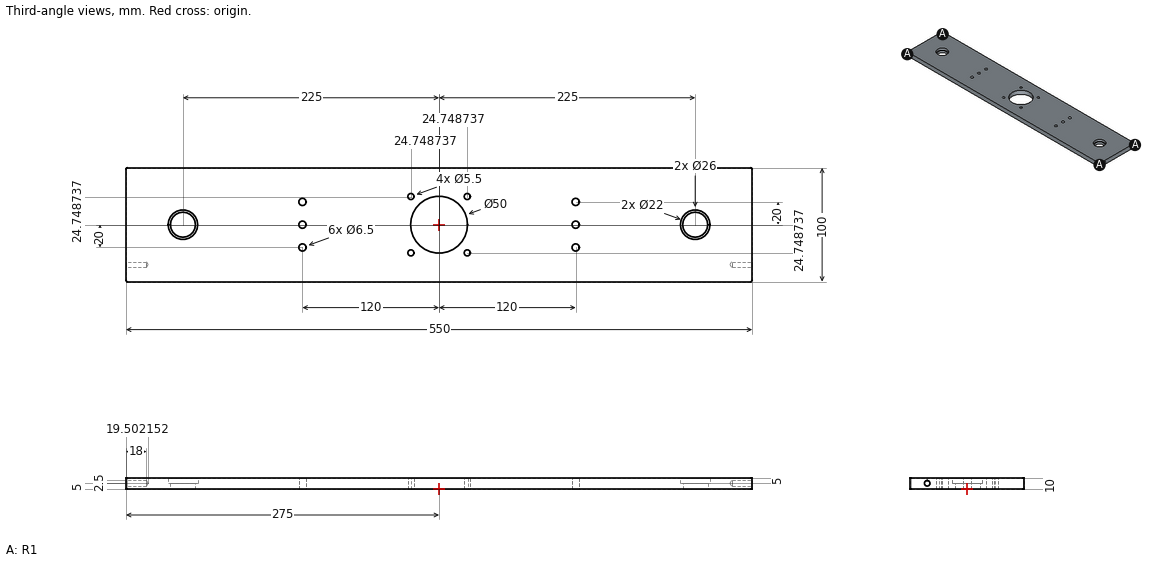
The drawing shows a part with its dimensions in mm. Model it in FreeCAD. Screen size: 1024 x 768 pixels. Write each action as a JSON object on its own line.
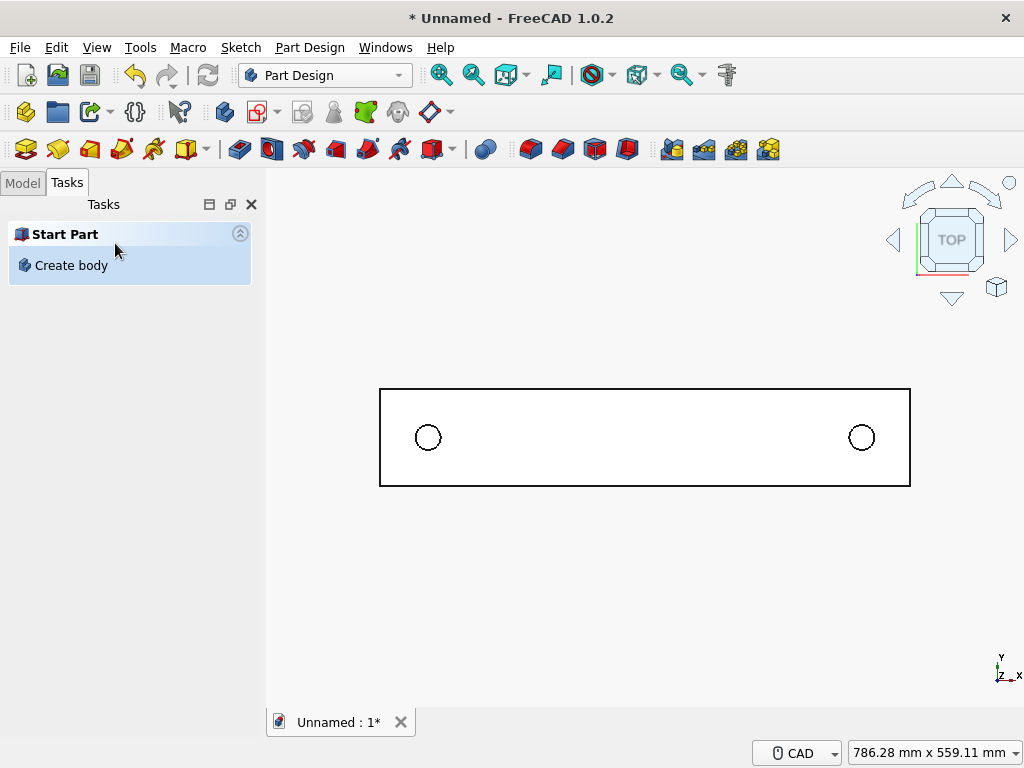
{"action": "left_click", "coordinate": [428, 437]}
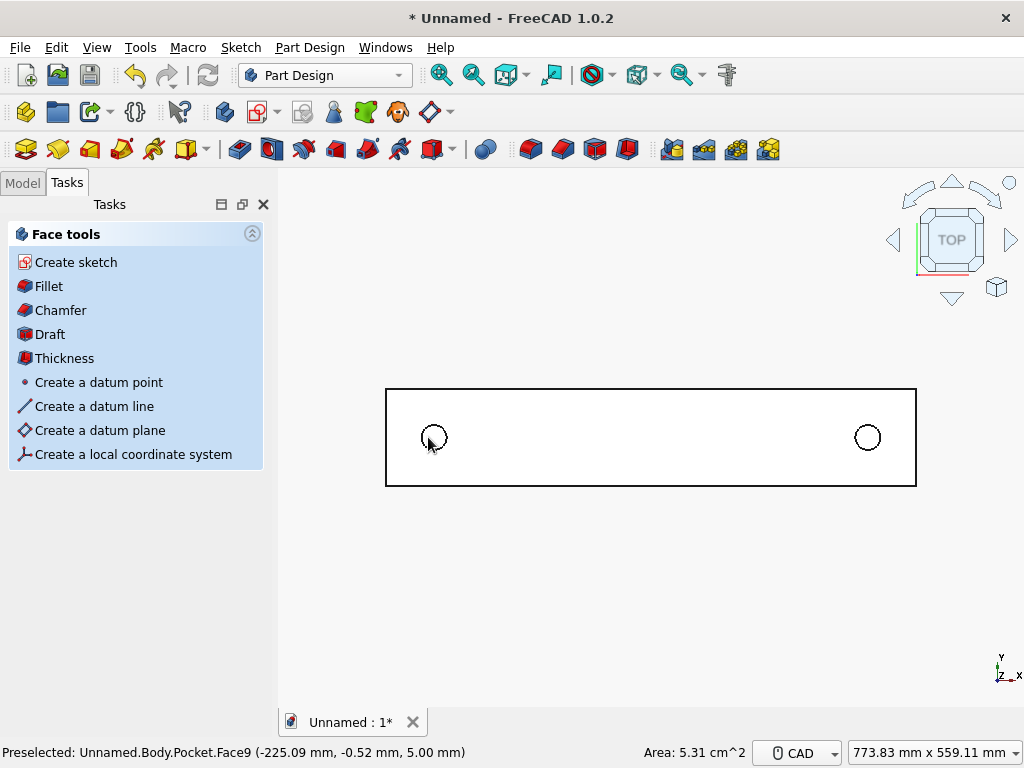
{"action": "left_click", "coordinate": [258, 112]}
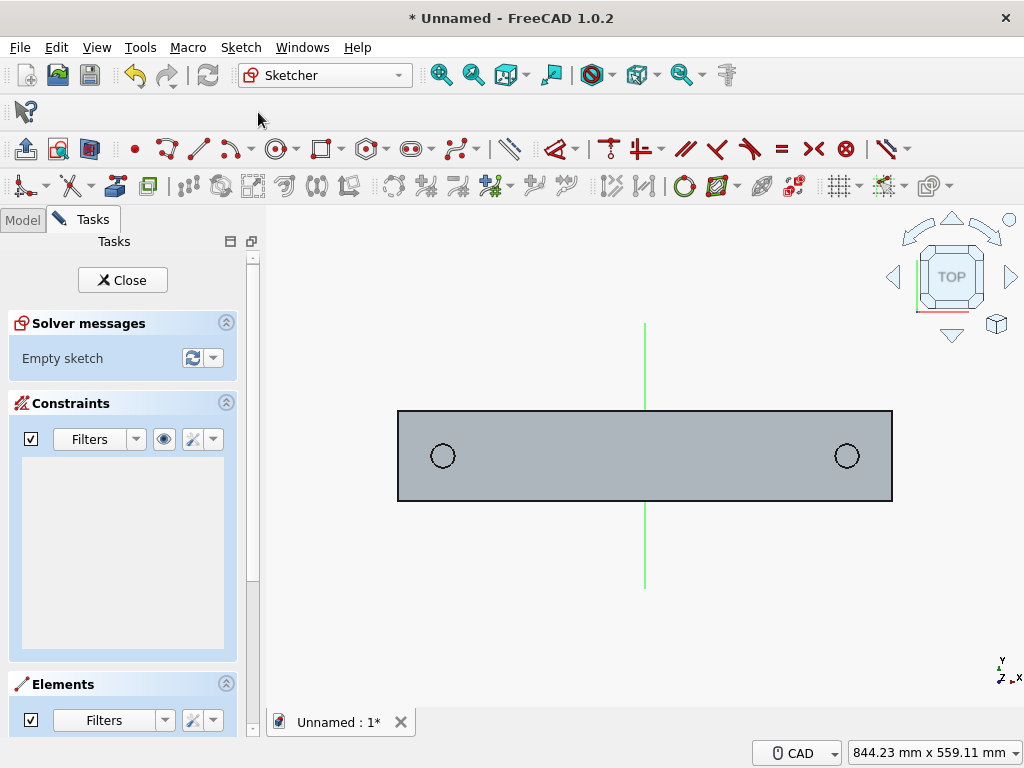
{"action": "scroll", "coordinate": [294, 456], "scroll_direction": "down", "scroll_amount": 1}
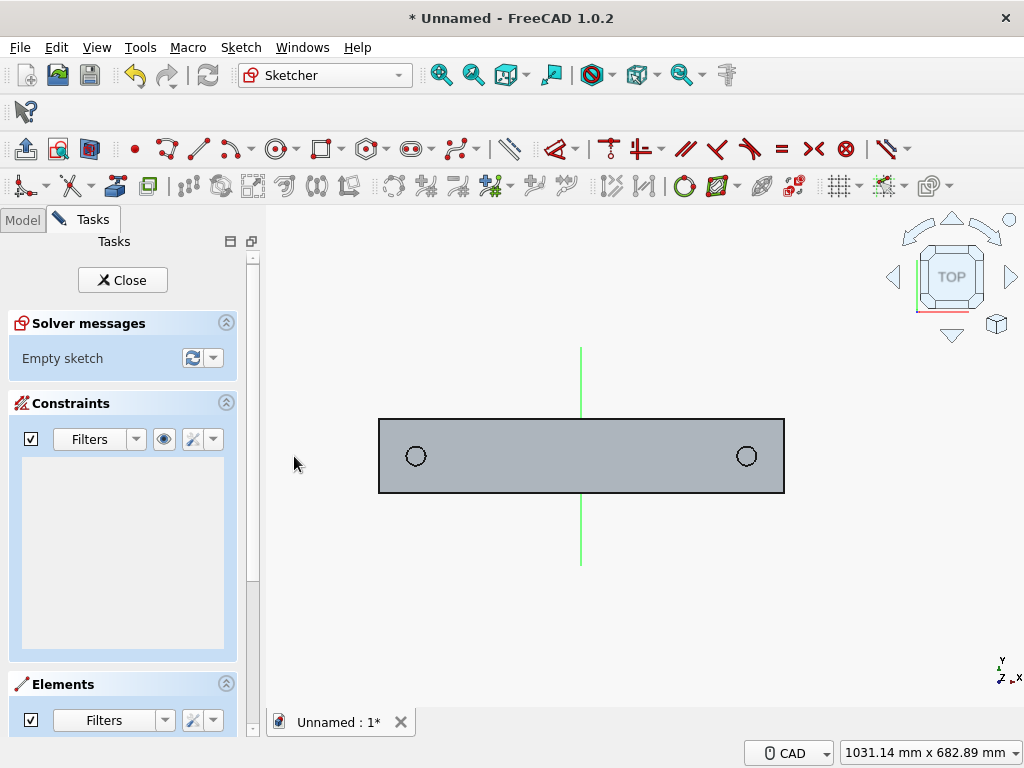
{"action": "key", "text": "g c"}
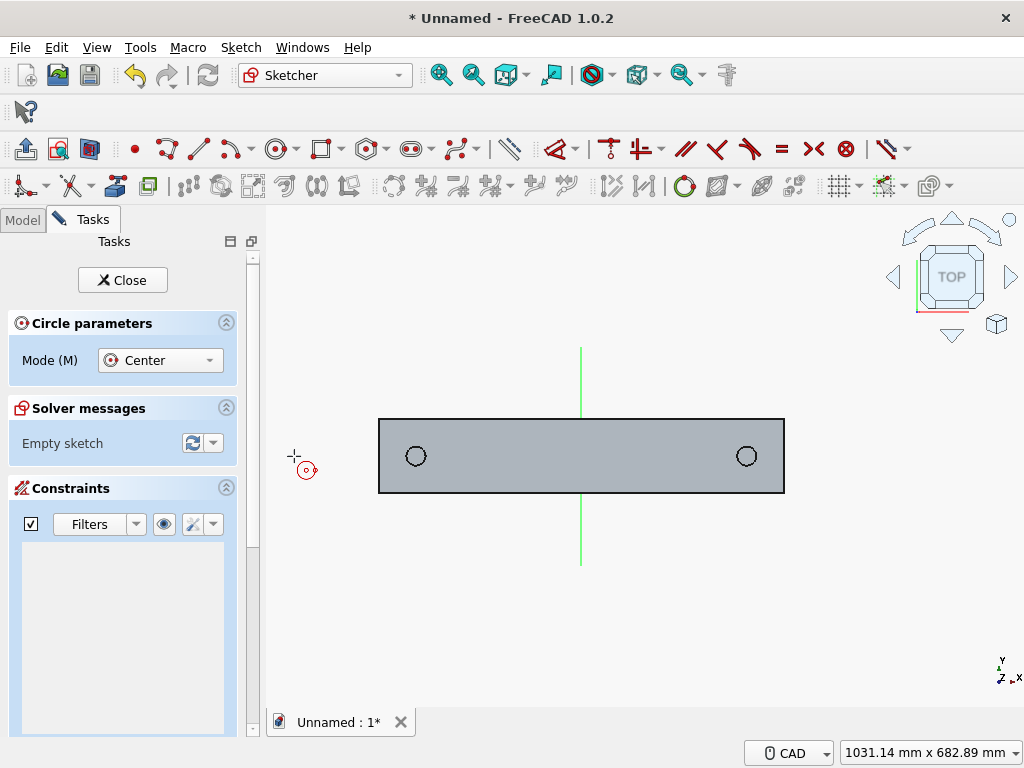
{"action": "scroll", "coordinate": [747, 456], "scroll_direction": "up", "scroll_amount": 6}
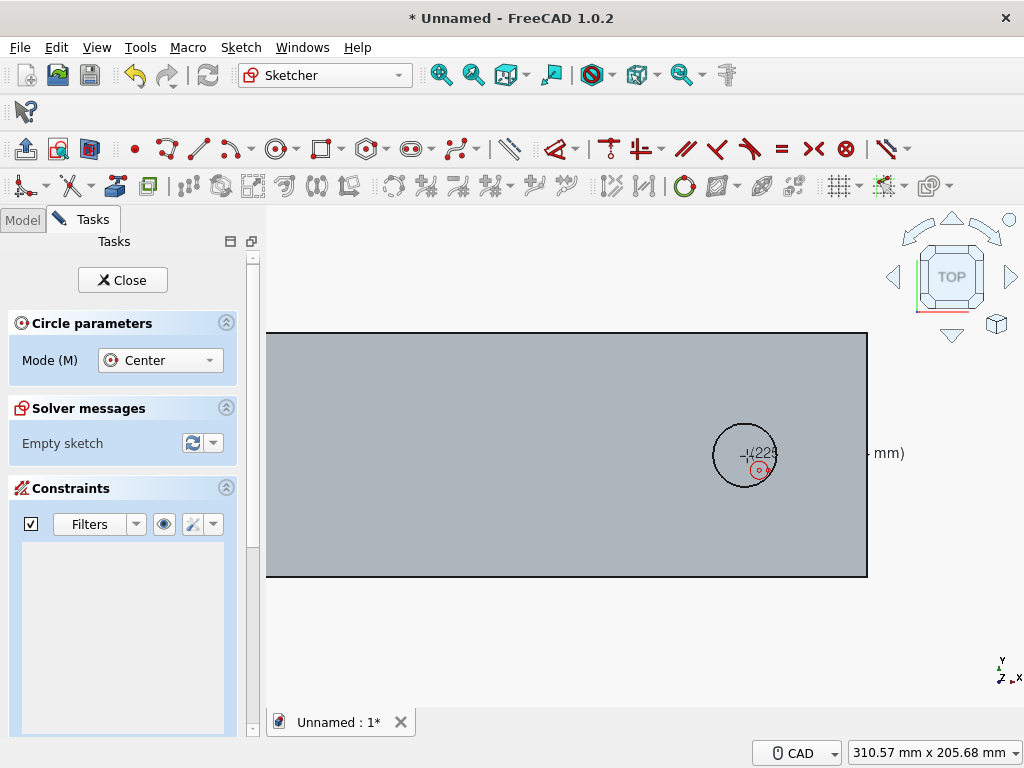
{"action": "left_click", "coordinate": [745, 455]}
{"action": "left_click", "coordinate": [764, 436]}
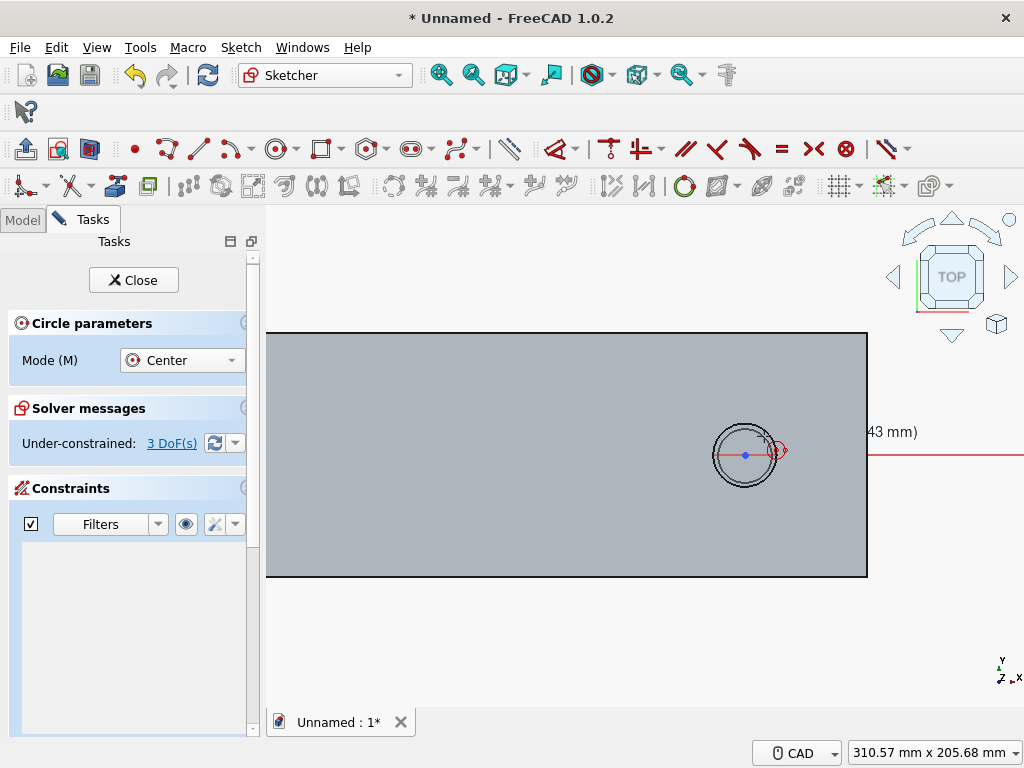
{"action": "scroll", "coordinate": [798, 457], "scroll_direction": "down", "scroll_amount": 5}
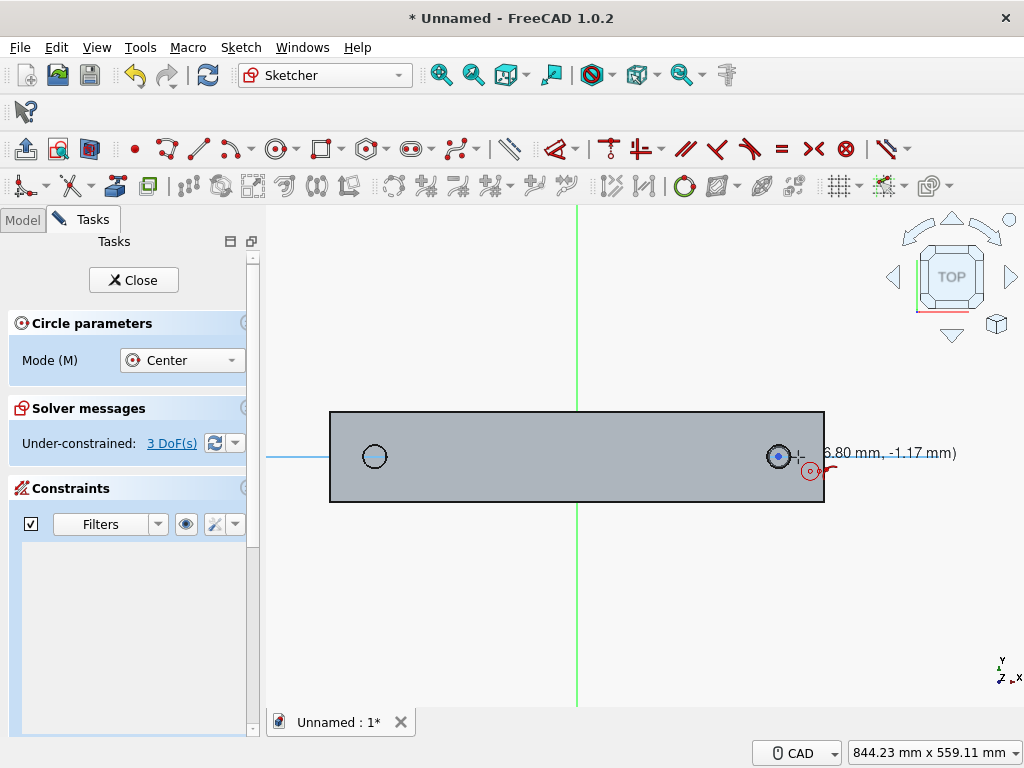
{"action": "scroll", "coordinate": [375, 457], "scroll_direction": "up", "scroll_amount": 5}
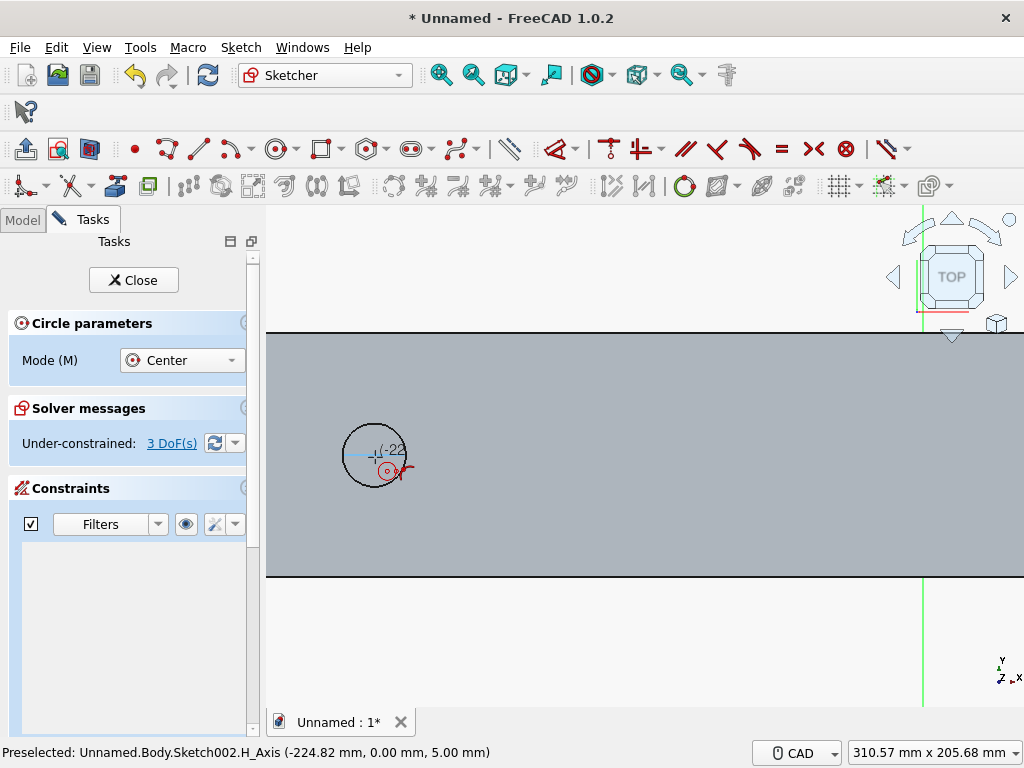
{"action": "left_click", "coordinate": [374, 455]}
{"action": "left_click", "coordinate": [393, 436]}
{"action": "key", "text": "Escape"}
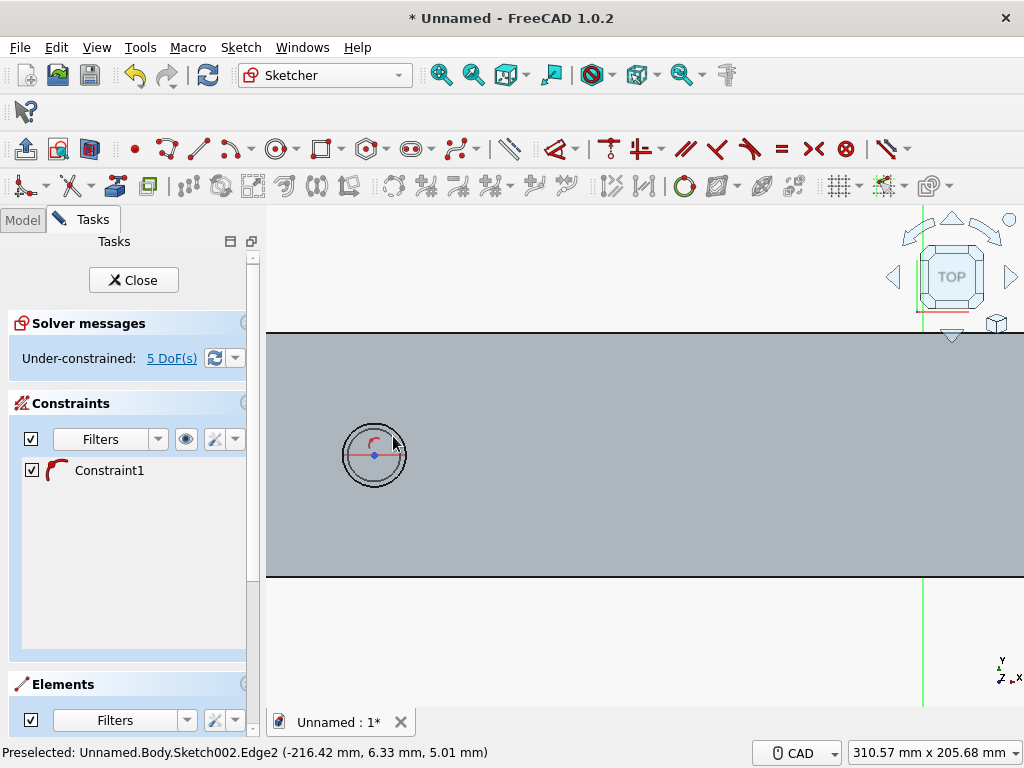
{"action": "scroll", "coordinate": [375, 457], "scroll_direction": "down", "scroll_amount": 5}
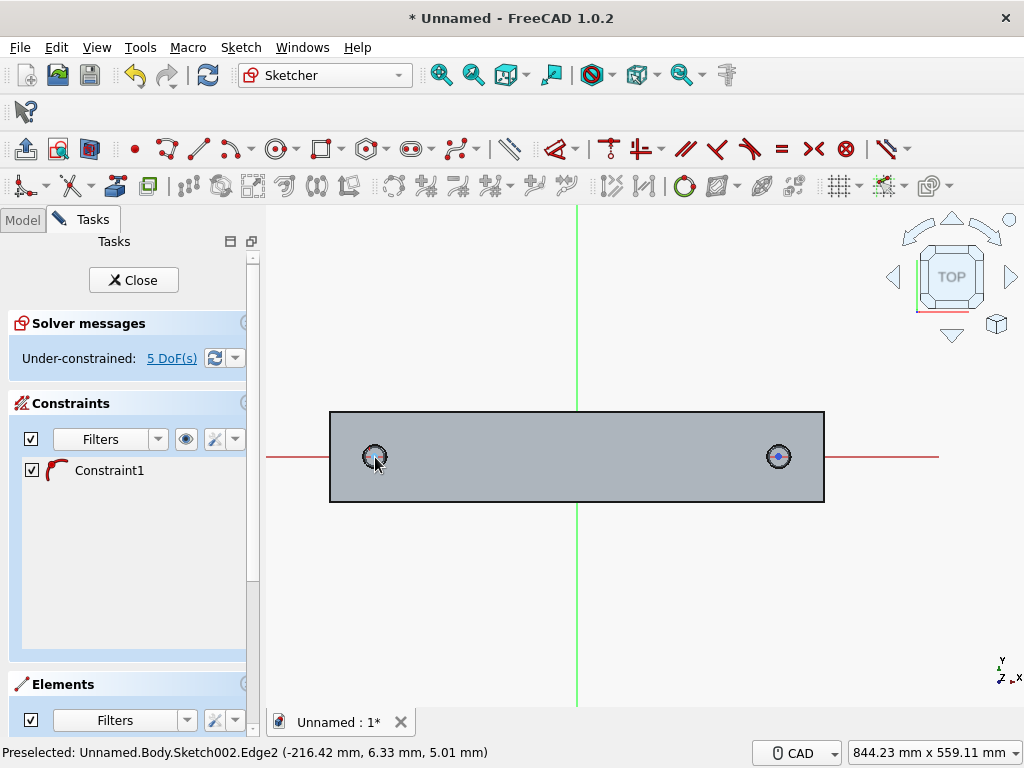
{"action": "scroll", "coordinate": [786, 450], "scroll_direction": "up", "scroll_amount": 4}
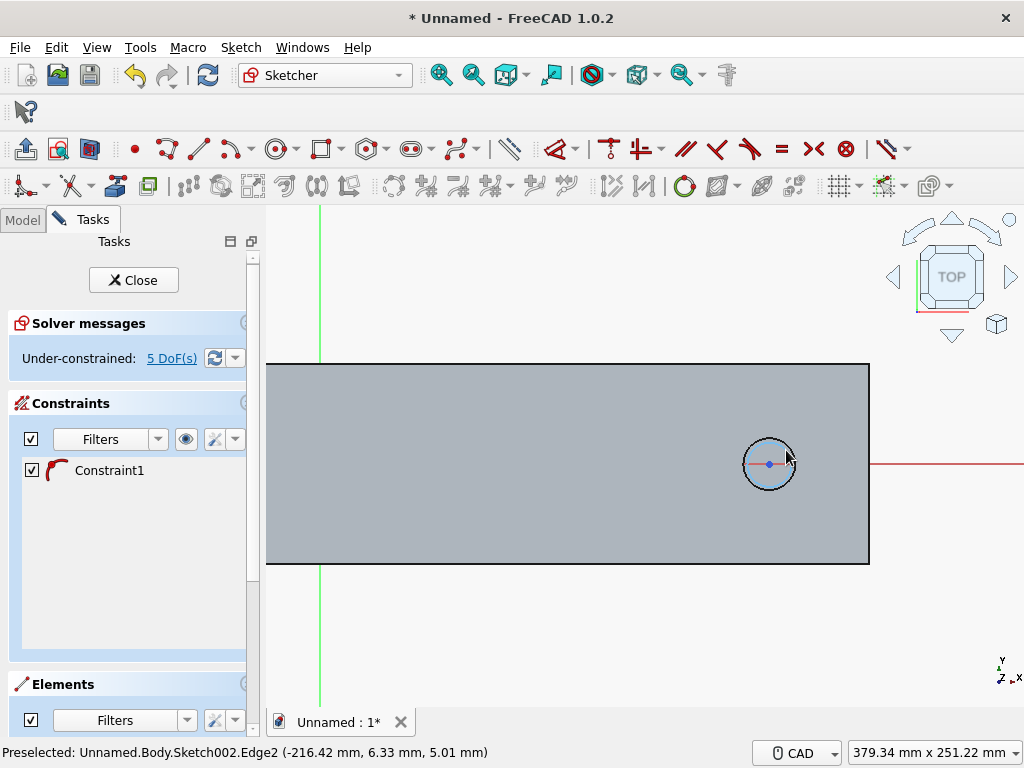
{"action": "left_click", "coordinate": [785, 449]}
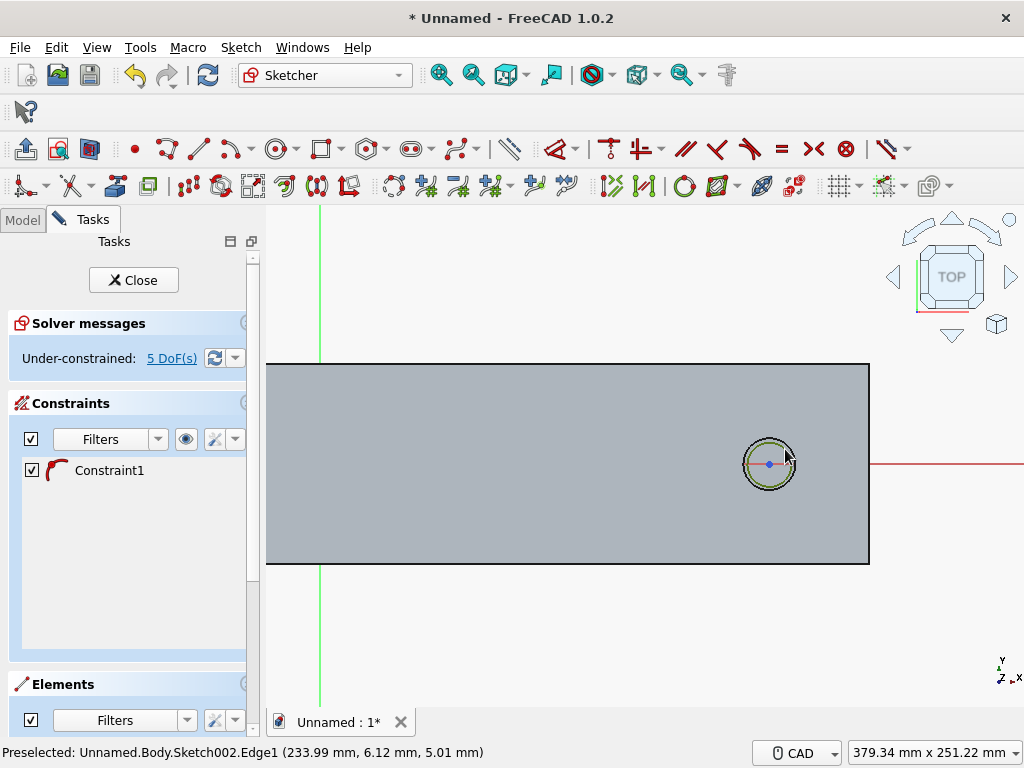
{"action": "scroll", "coordinate": [786, 449], "scroll_direction": "down", "scroll_amount": 4}